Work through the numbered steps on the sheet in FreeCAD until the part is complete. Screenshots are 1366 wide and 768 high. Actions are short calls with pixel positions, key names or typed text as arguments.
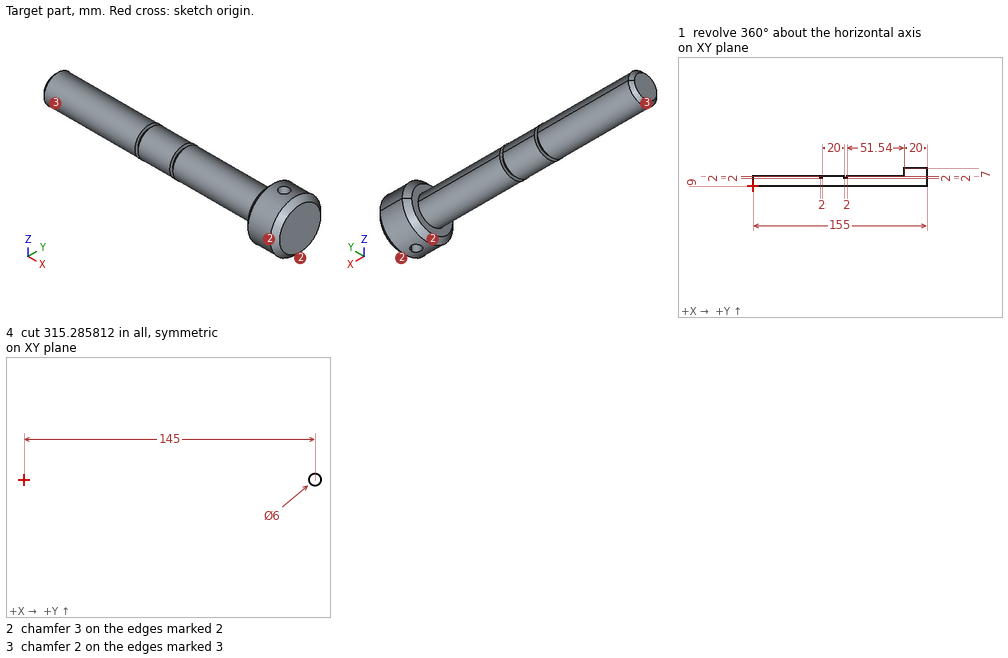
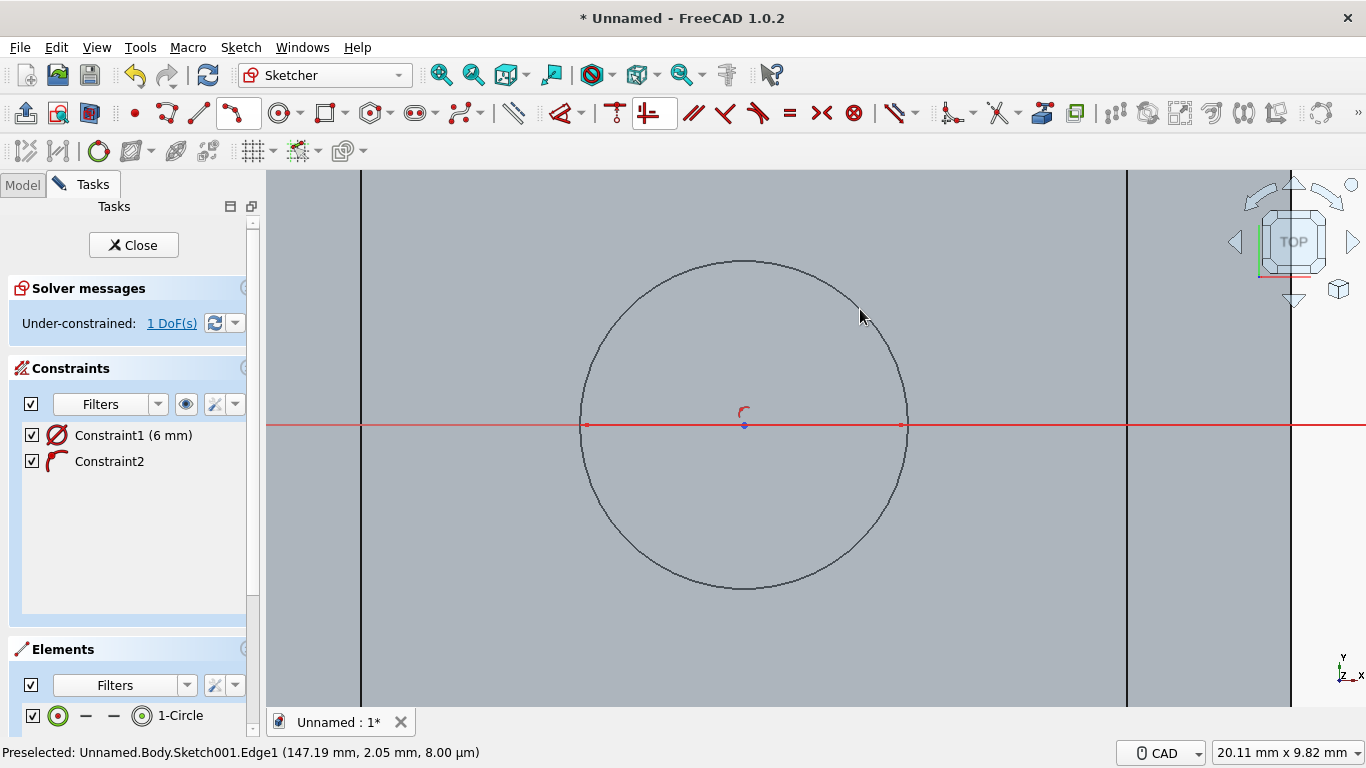
click(560, 114)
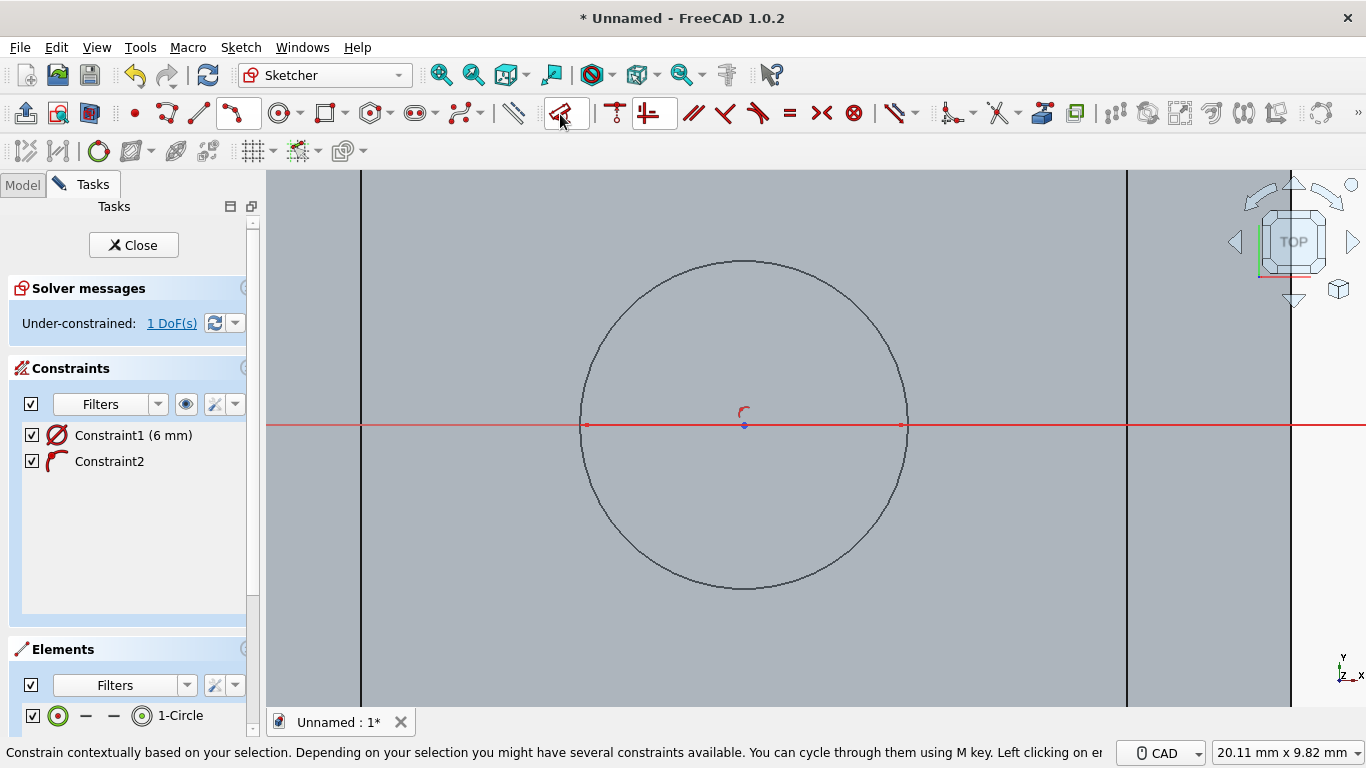
click(744, 425)
click(519, 459)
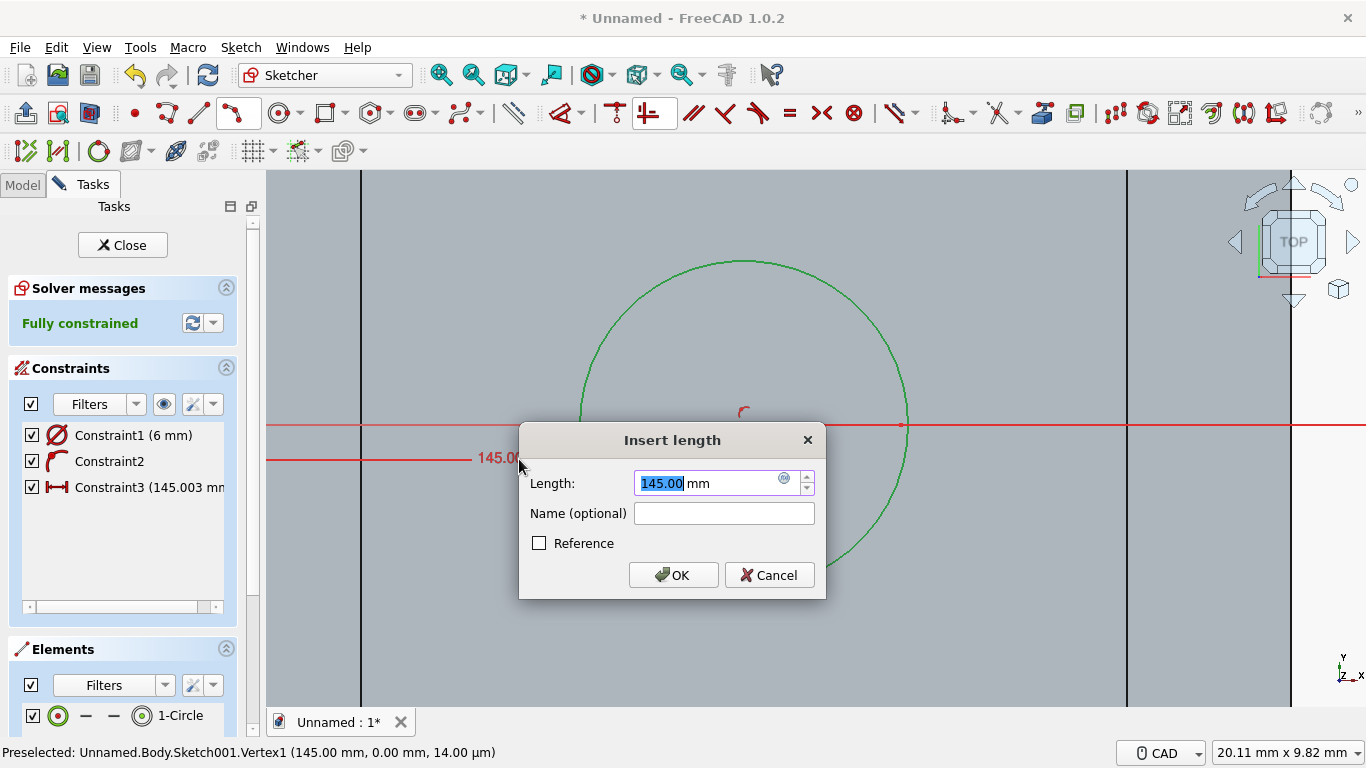
text(145)
key(Return)
key(Escape)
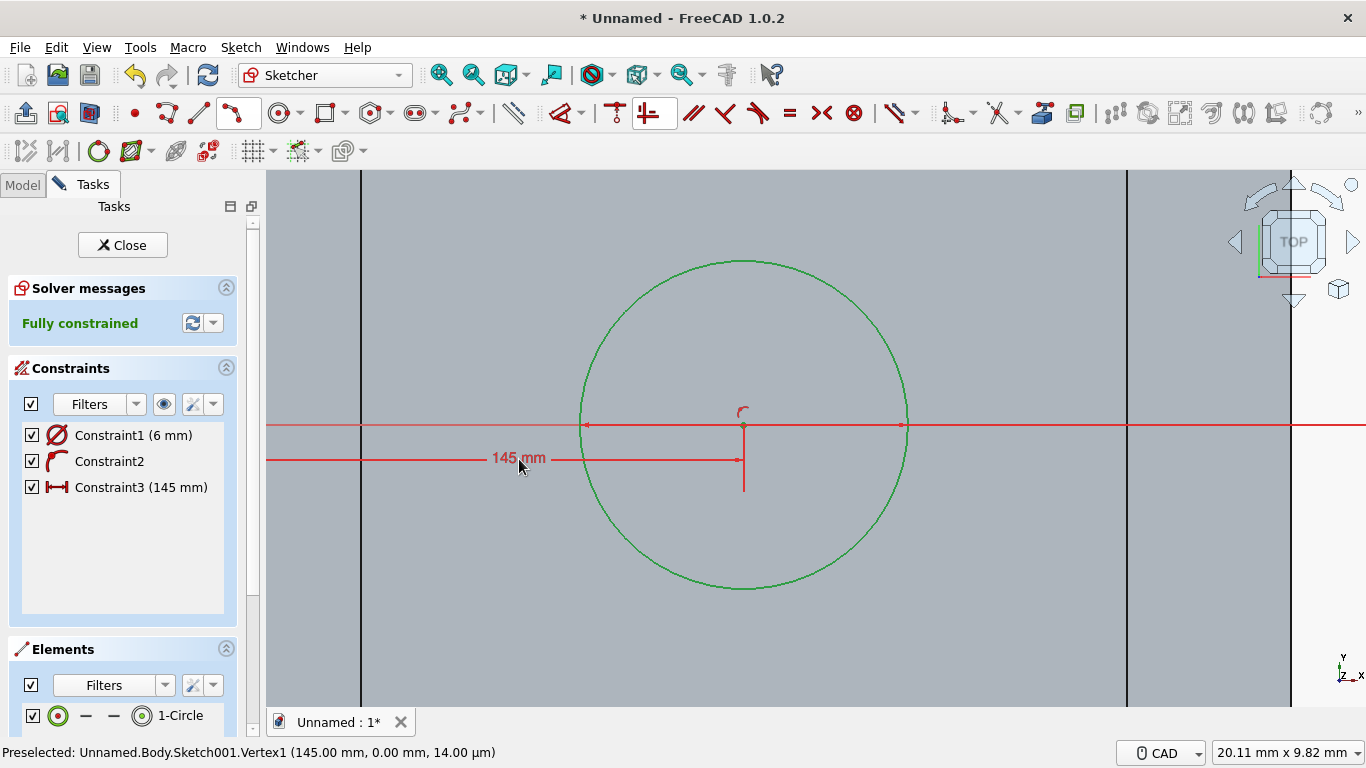
click(123, 245)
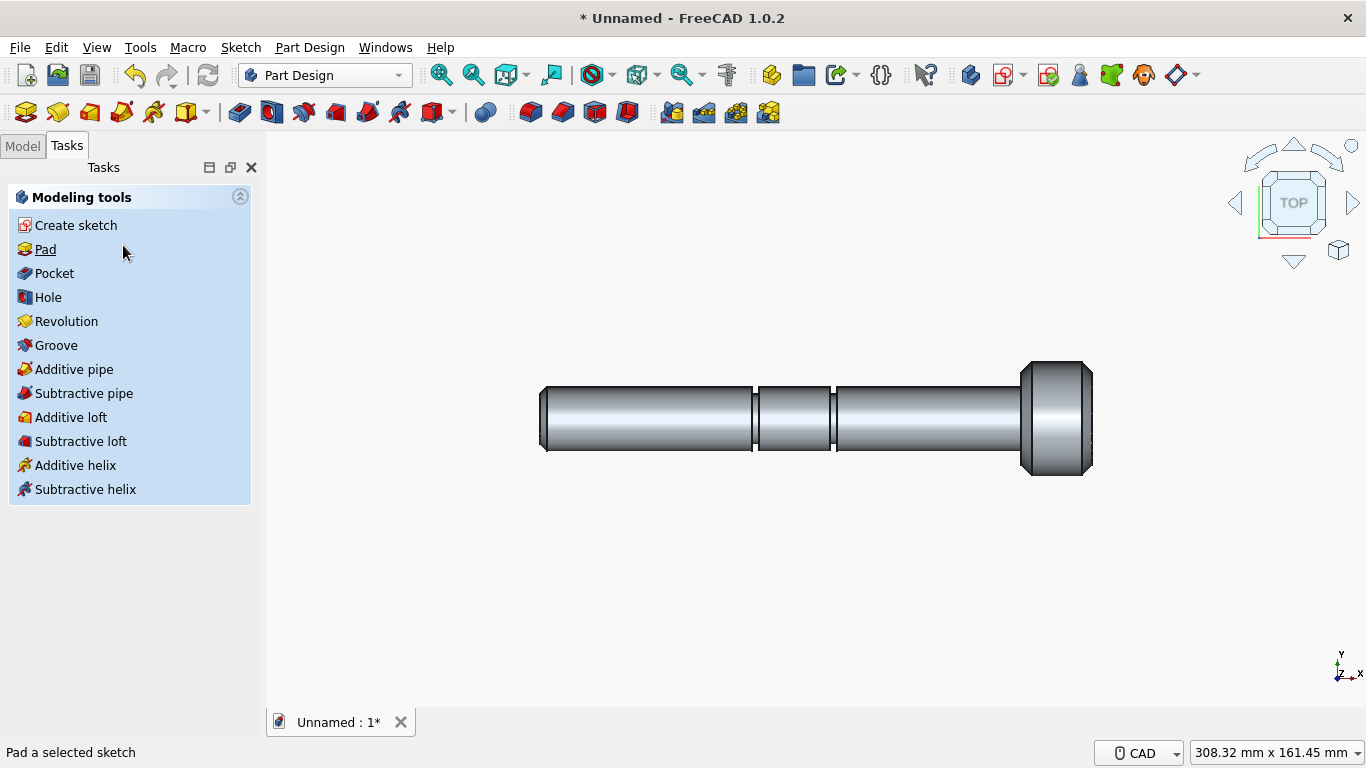
click(240, 112)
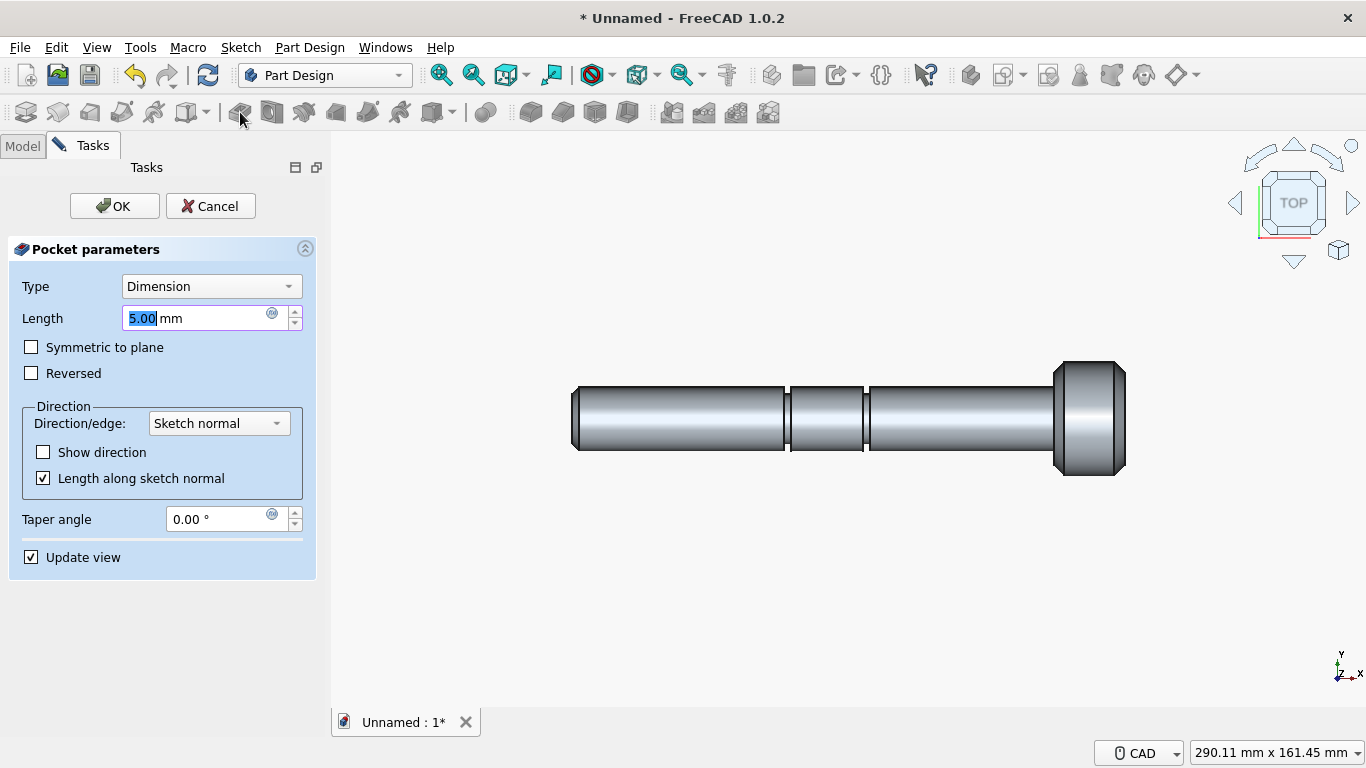
text(315.285812)
key(Tab)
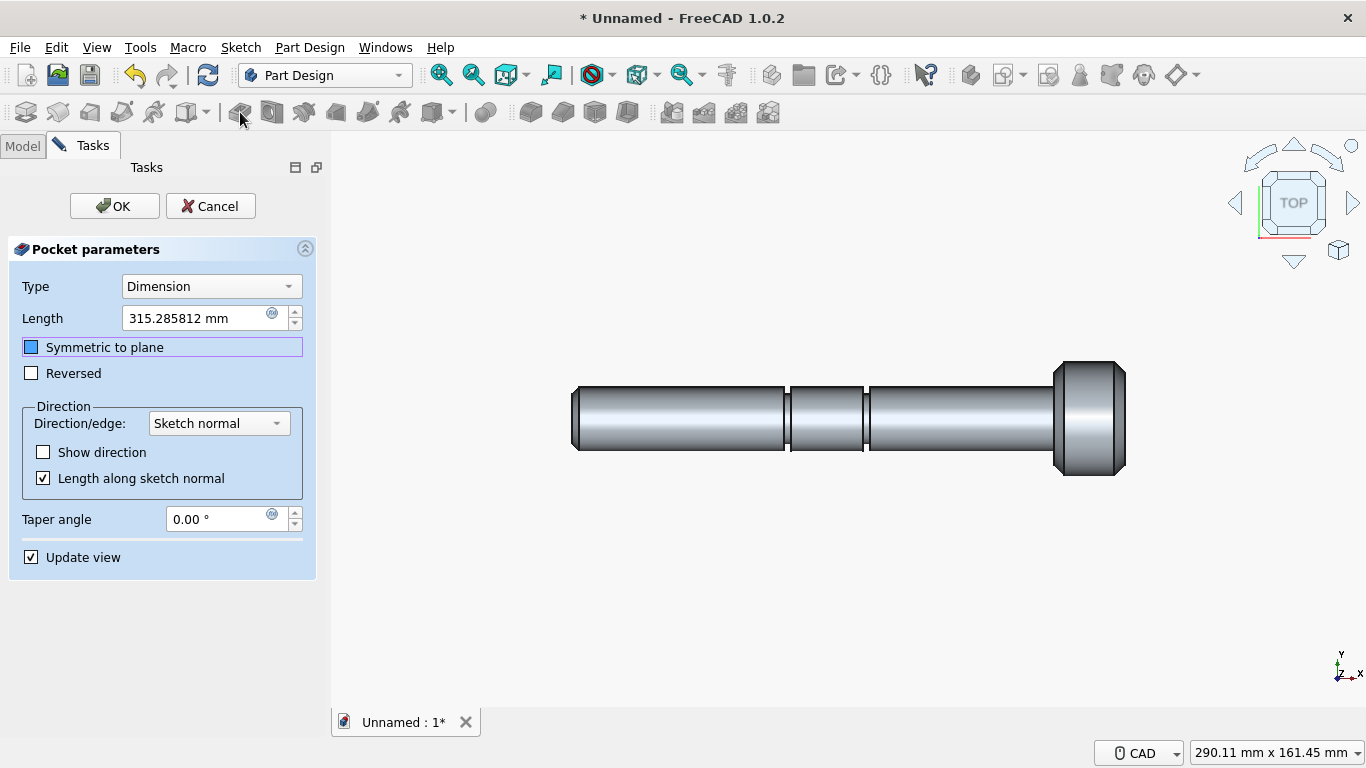
click(30, 347)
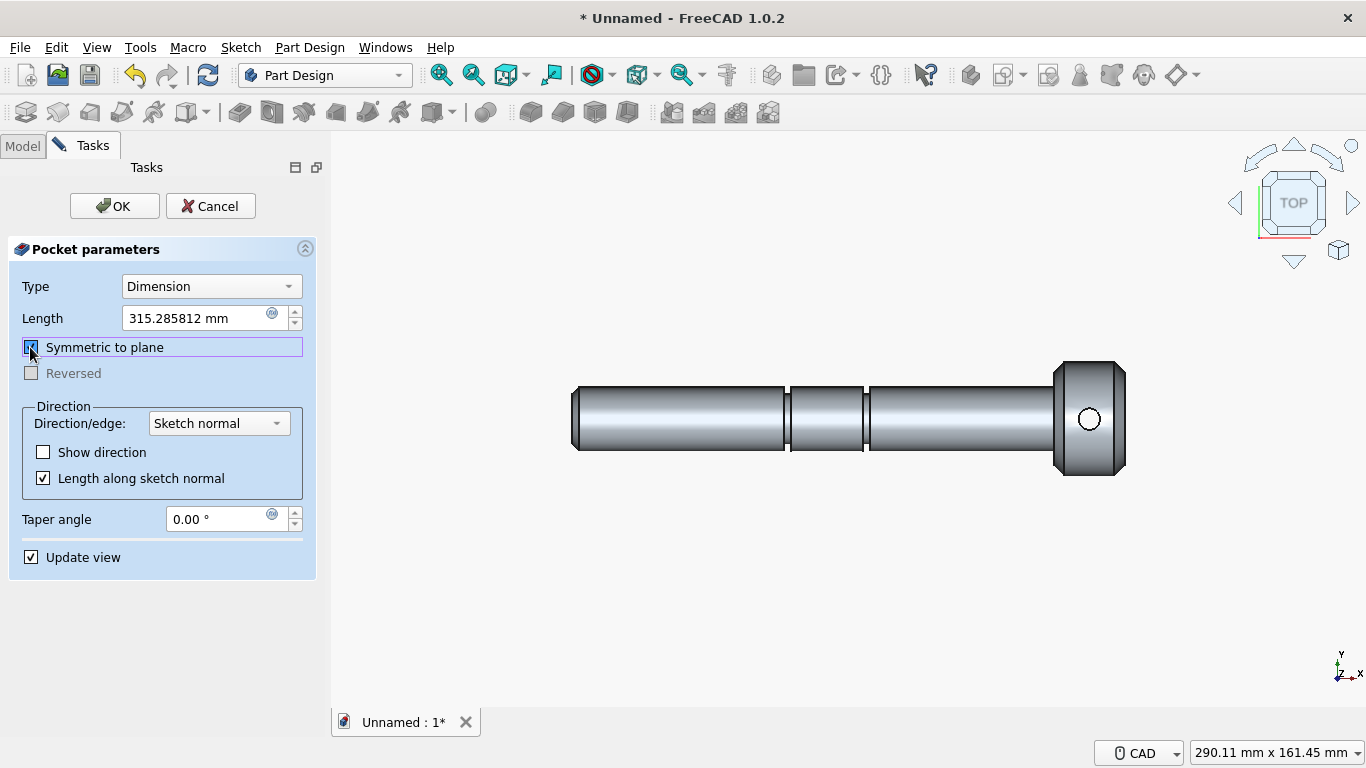
click(115, 206)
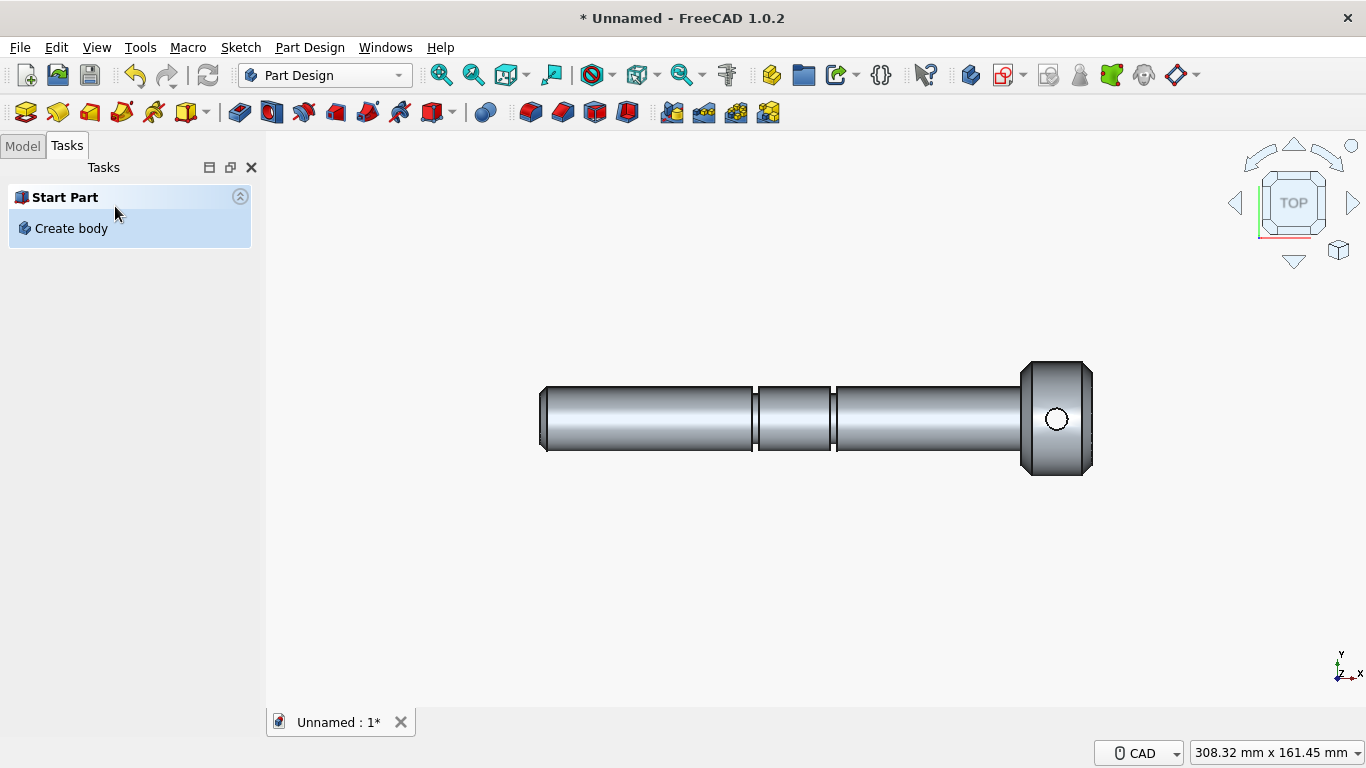
key(0)